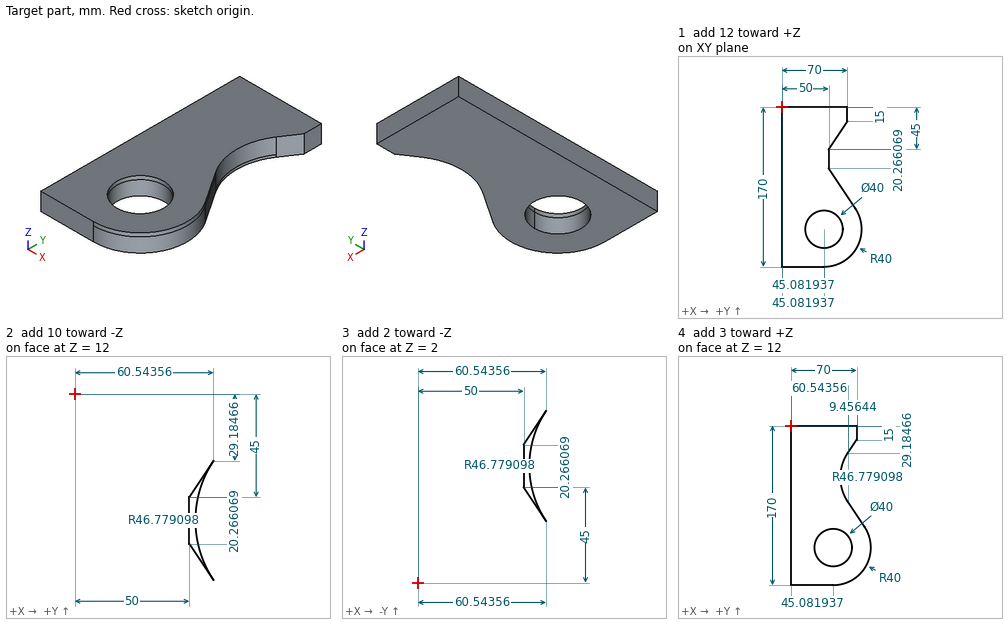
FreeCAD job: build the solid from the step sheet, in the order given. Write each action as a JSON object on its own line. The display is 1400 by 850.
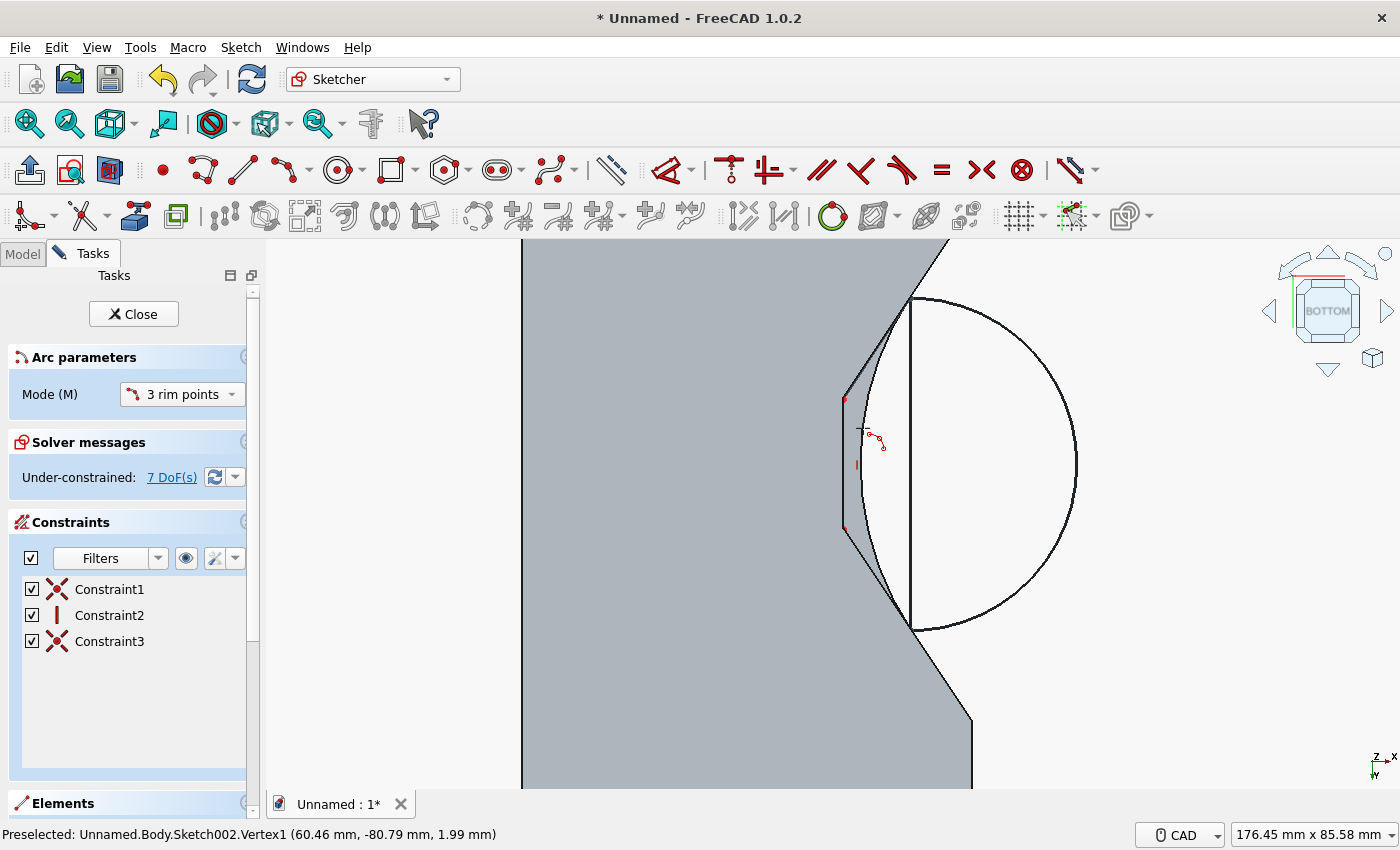
{"action": "left_click", "coordinate": [863, 428]}
{"action": "key", "text": "Escape"}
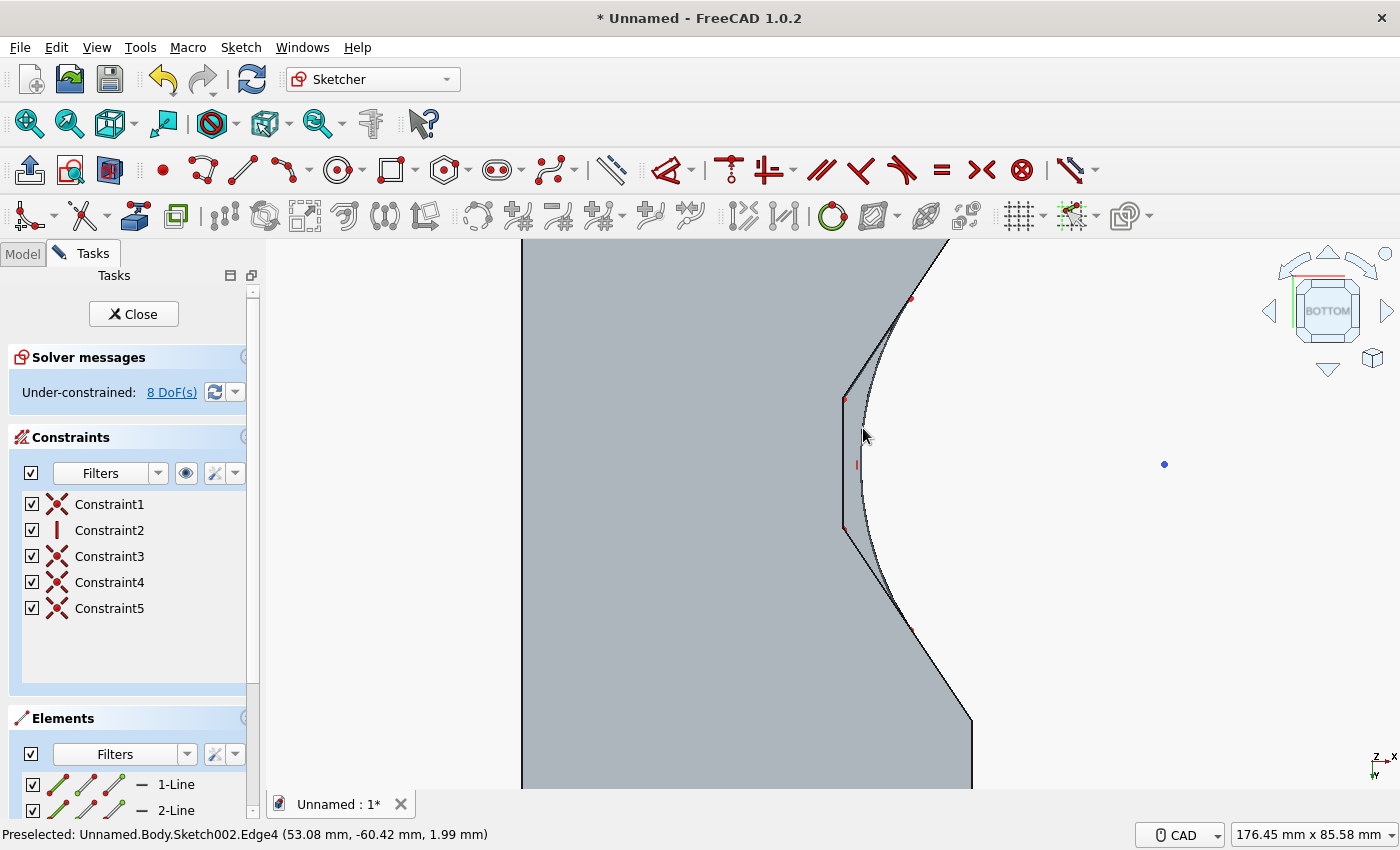
{"action": "left_click", "coordinate": [863, 369]}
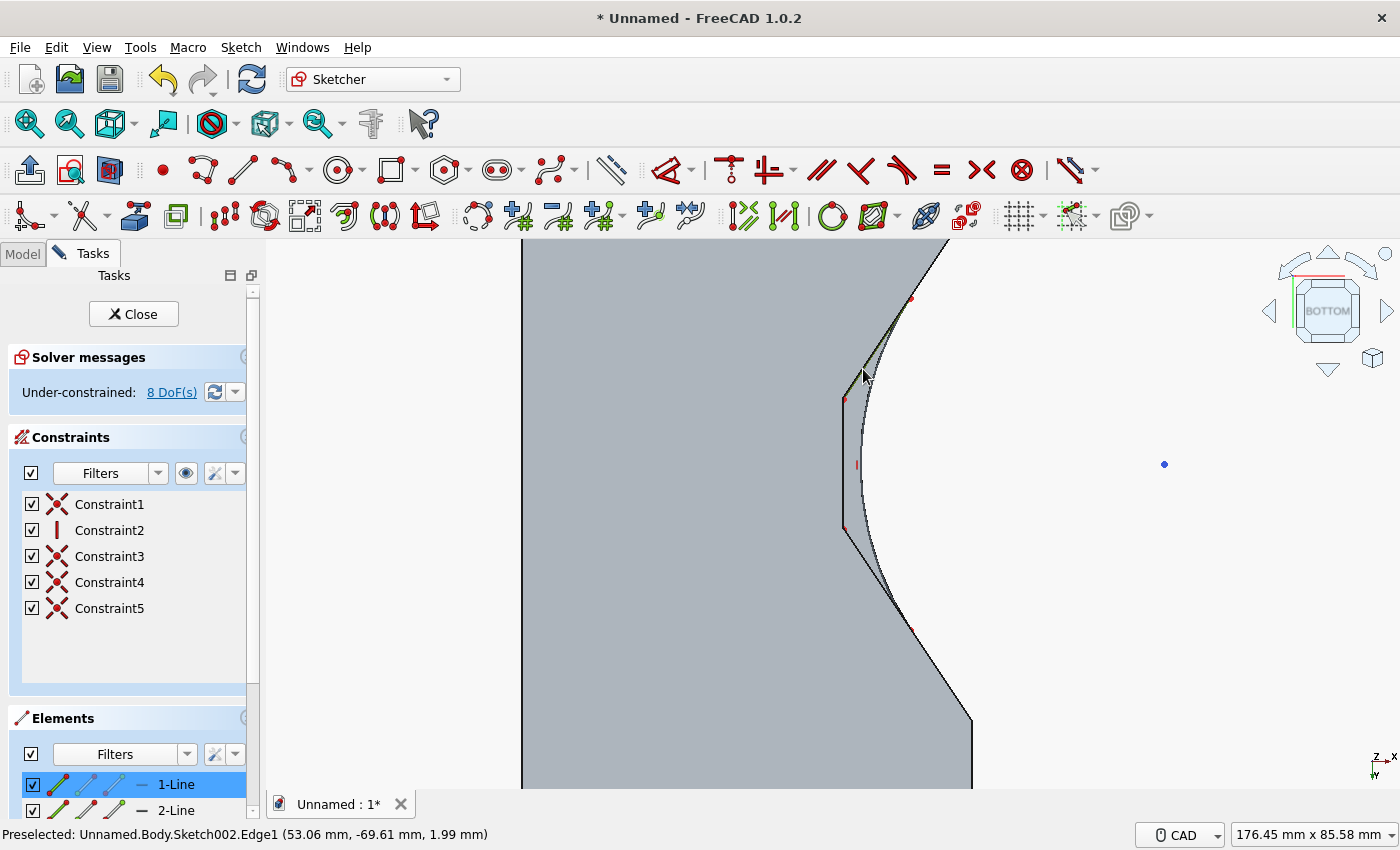
{"action": "left_click", "coordinate": [869, 395]}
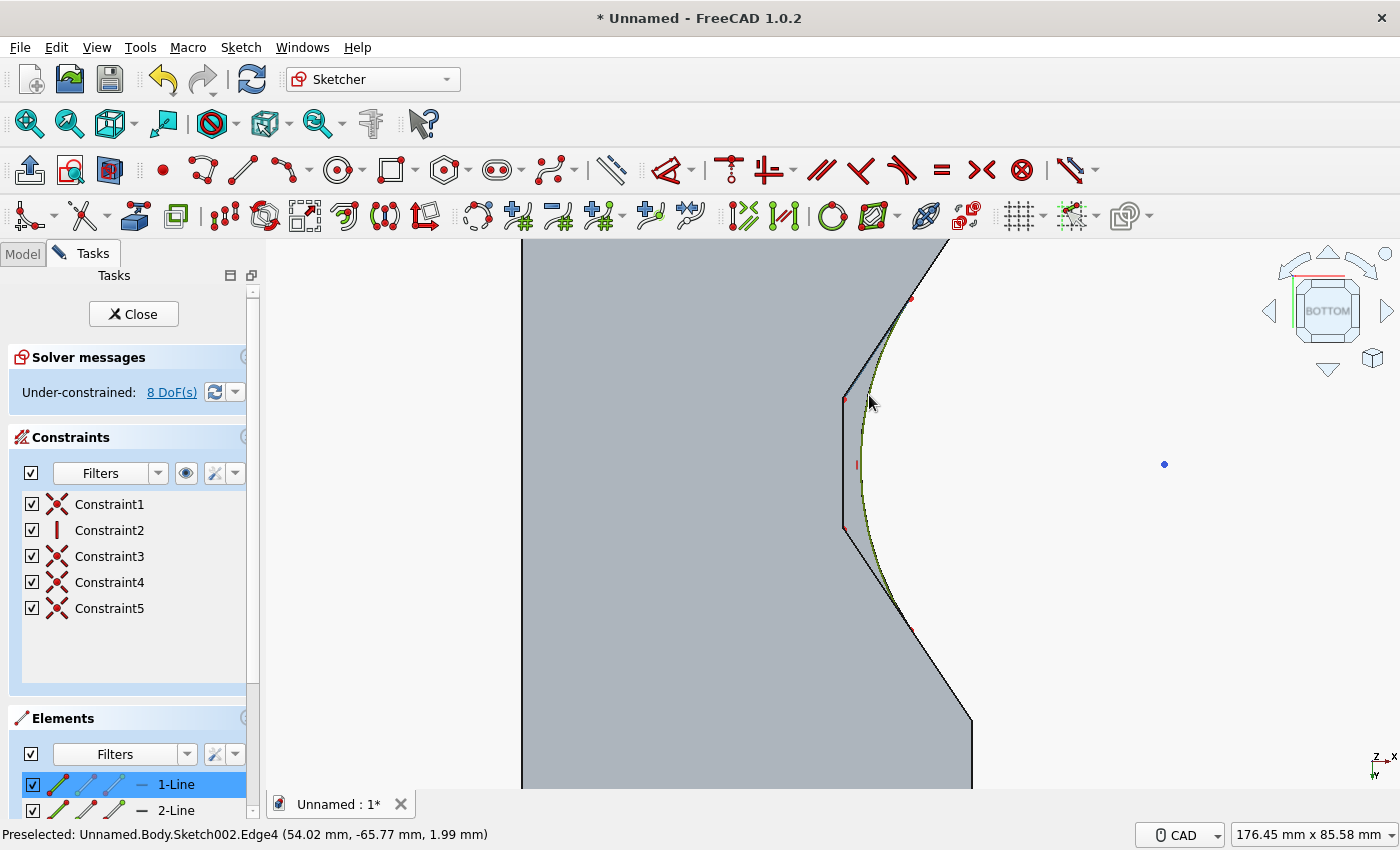
{"action": "left_click", "coordinate": [902, 170]}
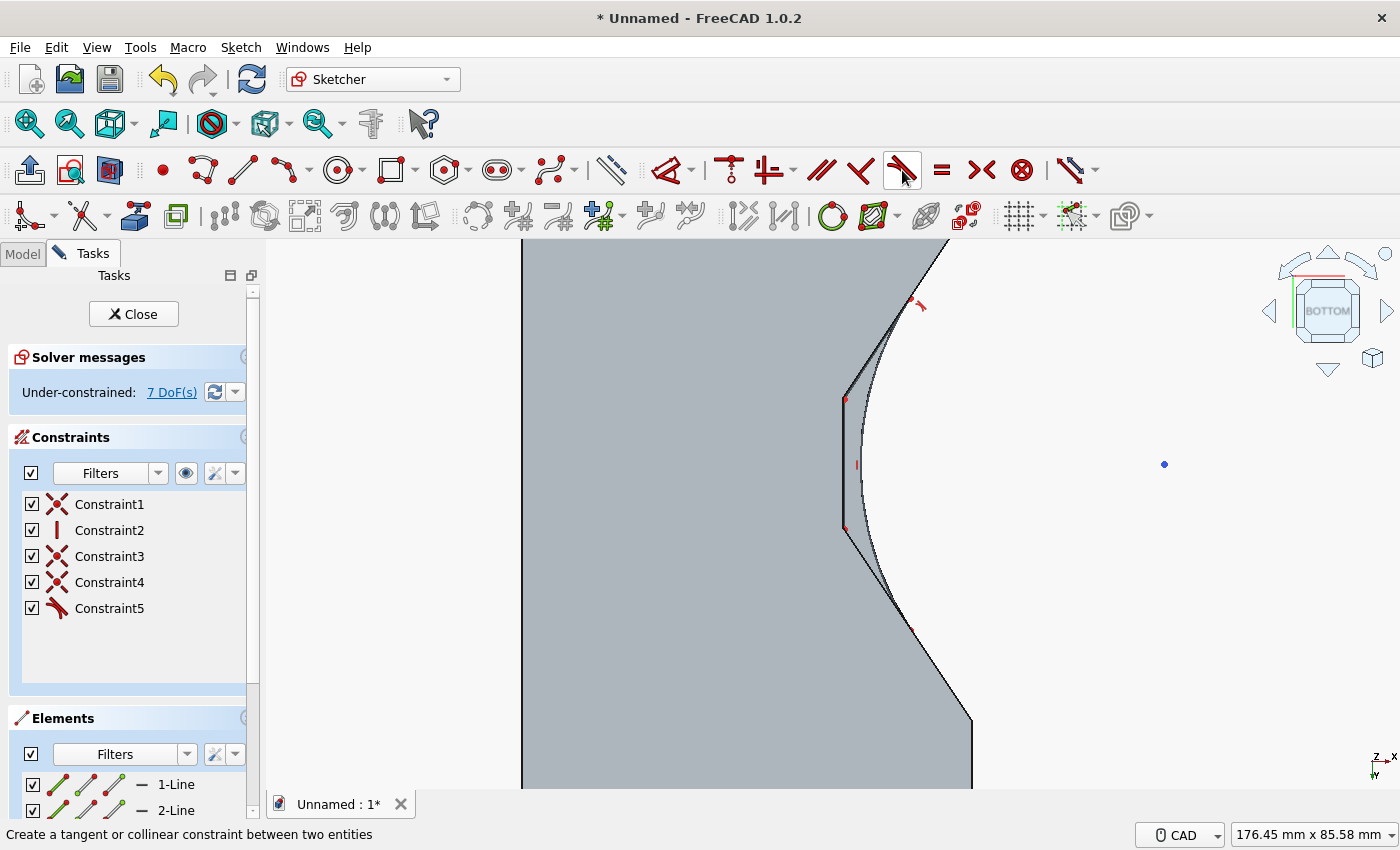
{"action": "left_click", "coordinate": [864, 560]}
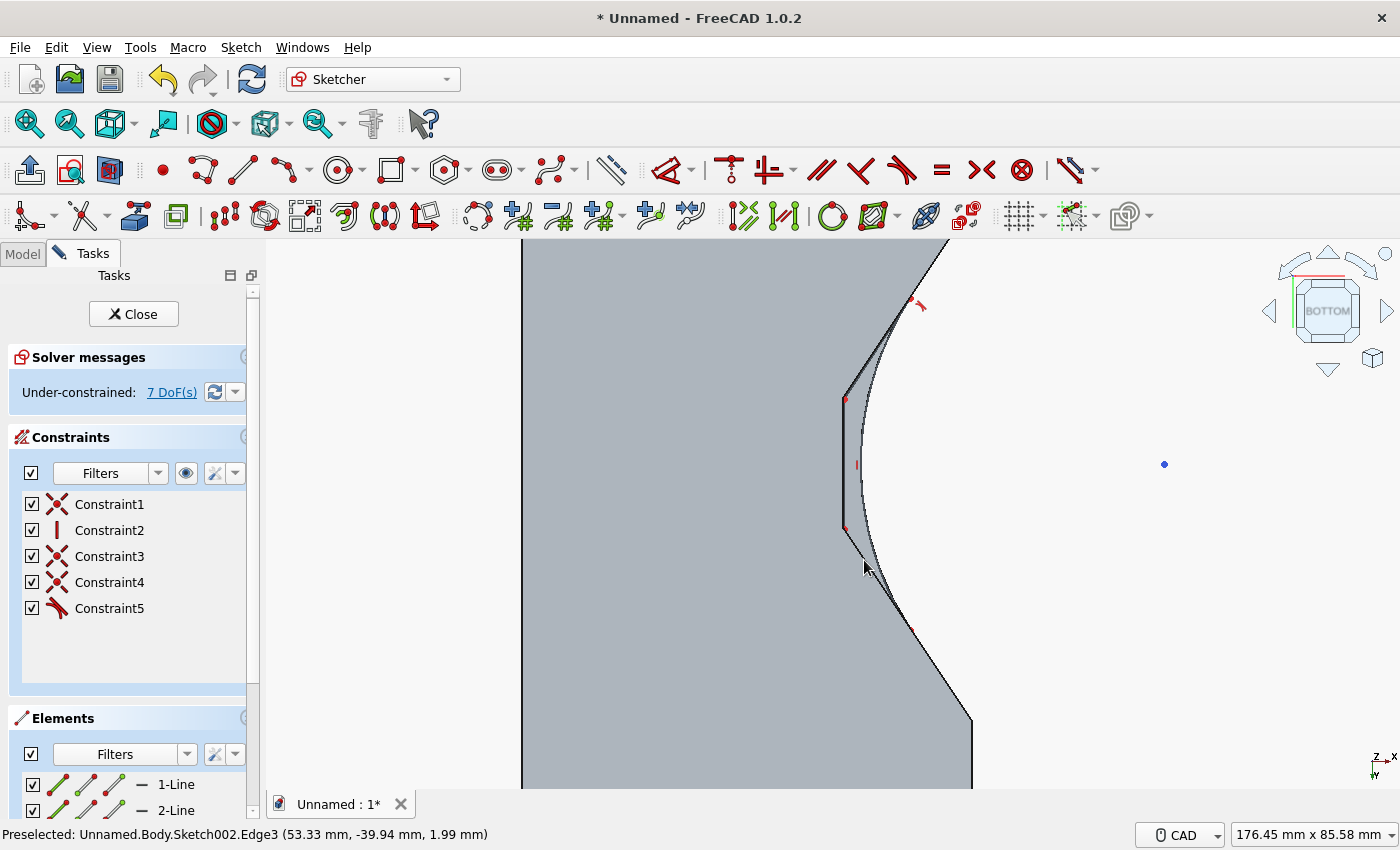
{"action": "left_click", "coordinate": [869, 395]}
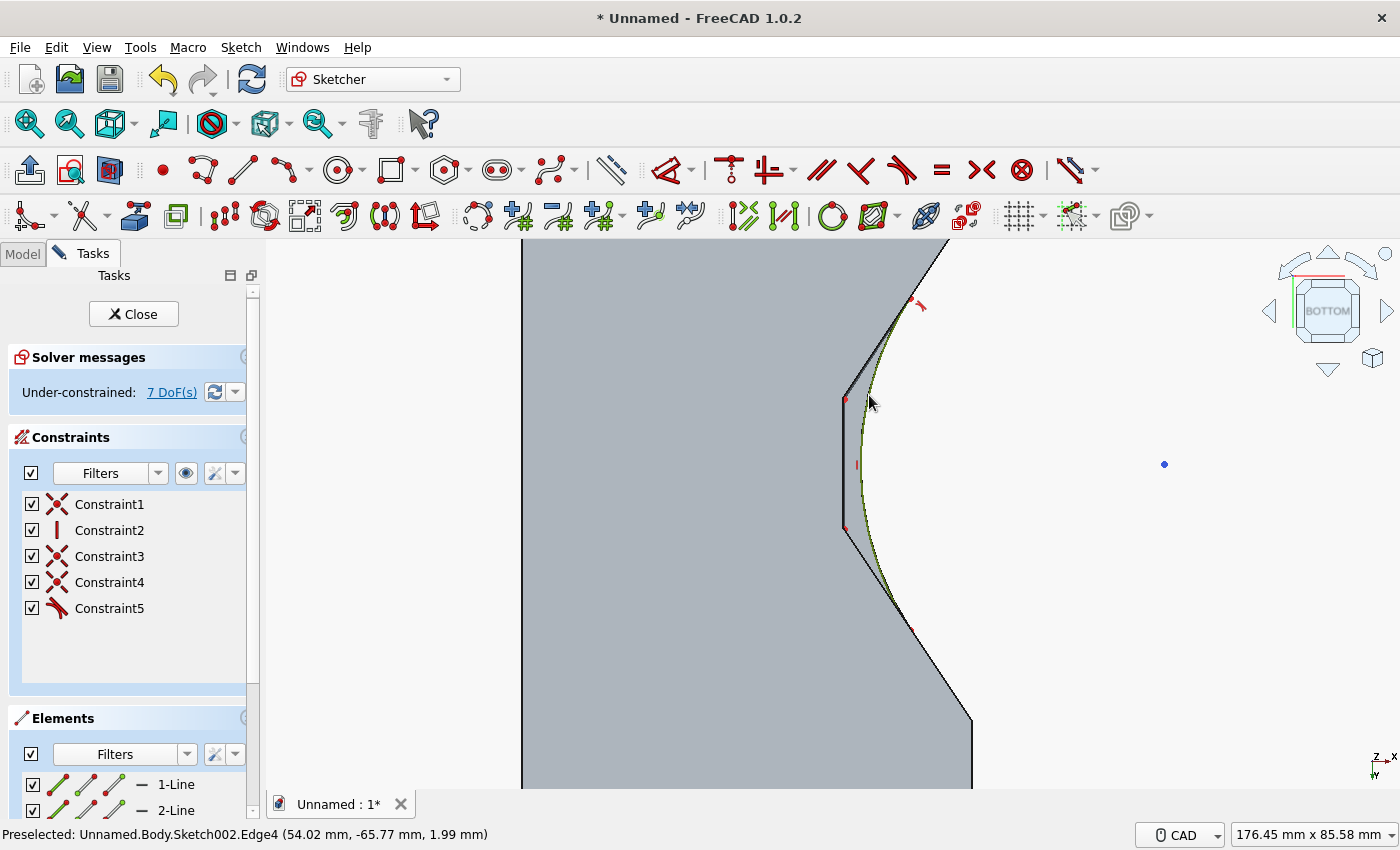
{"action": "left_click", "coordinate": [902, 170]}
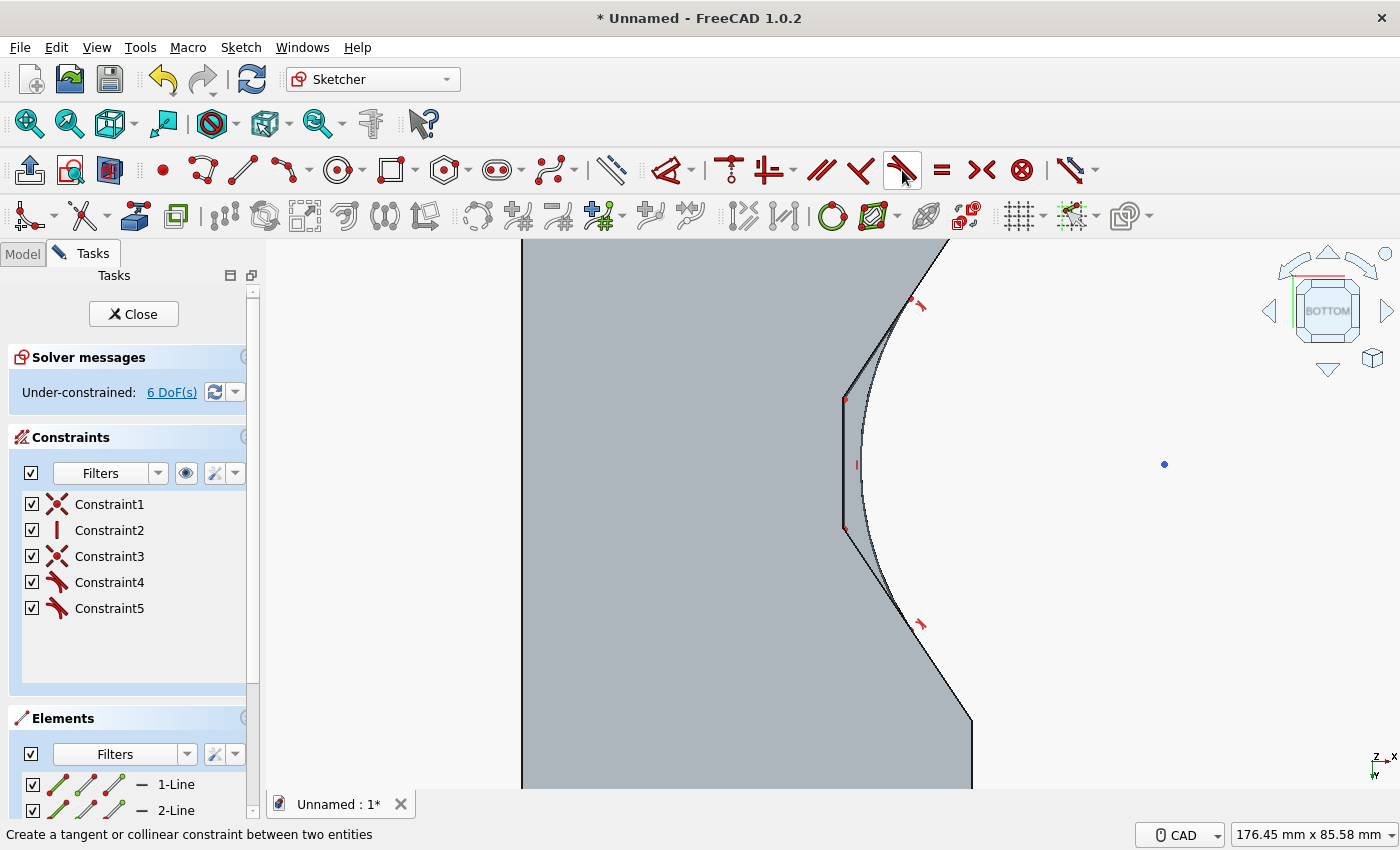
{"action": "left_click", "coordinate": [666, 170]}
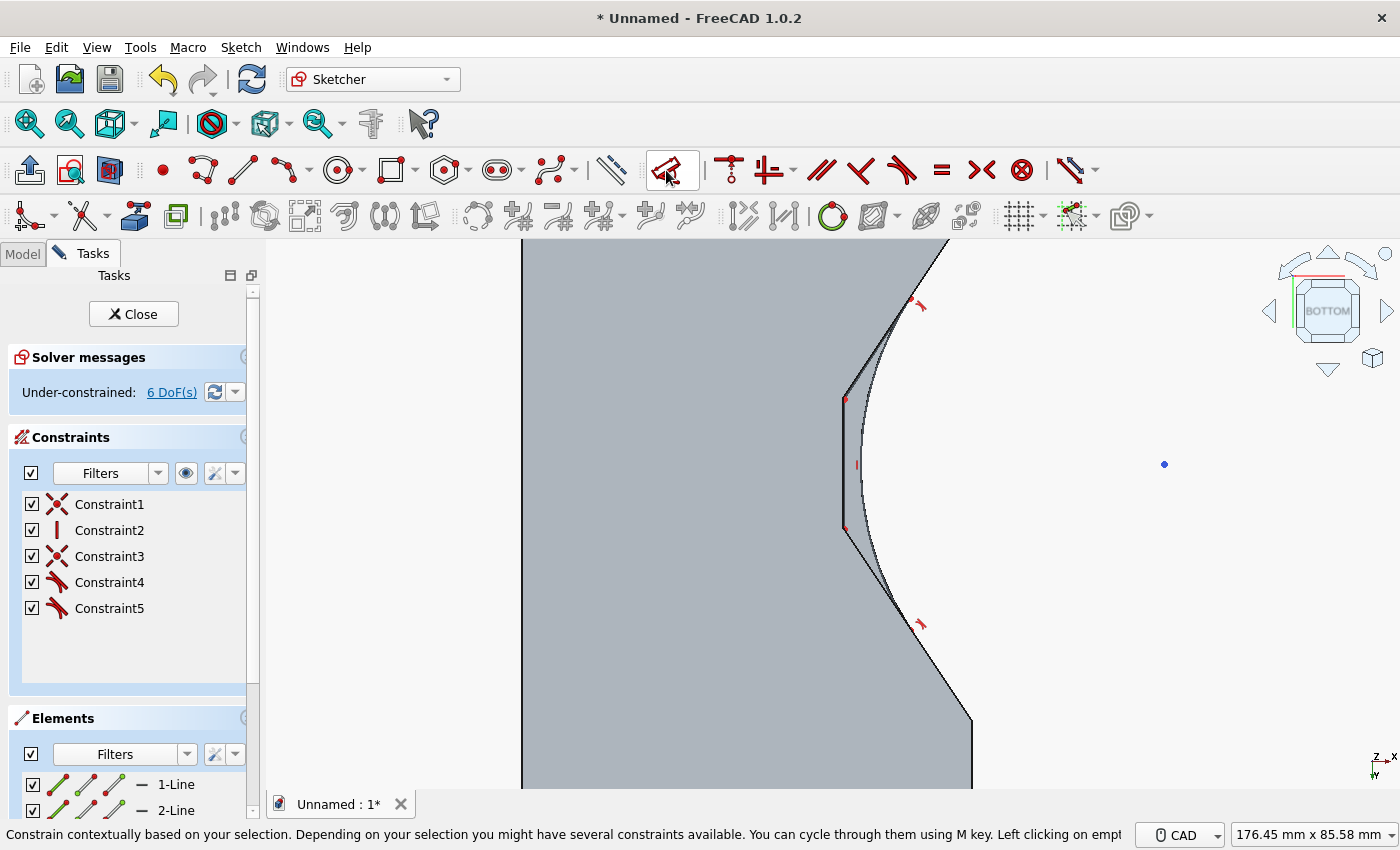
{"action": "left_click", "coordinate": [869, 395]}
{"action": "left_click", "coordinate": [841, 554]}